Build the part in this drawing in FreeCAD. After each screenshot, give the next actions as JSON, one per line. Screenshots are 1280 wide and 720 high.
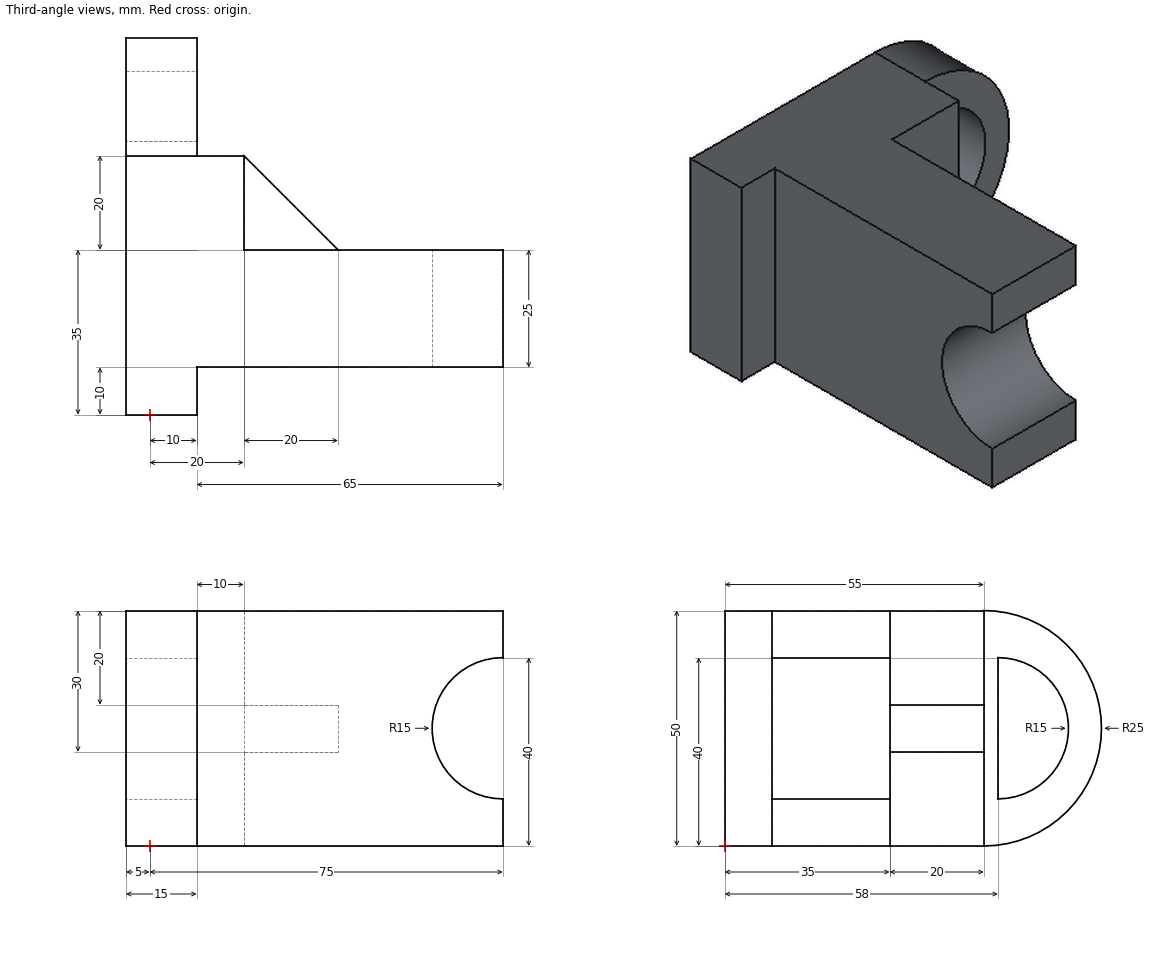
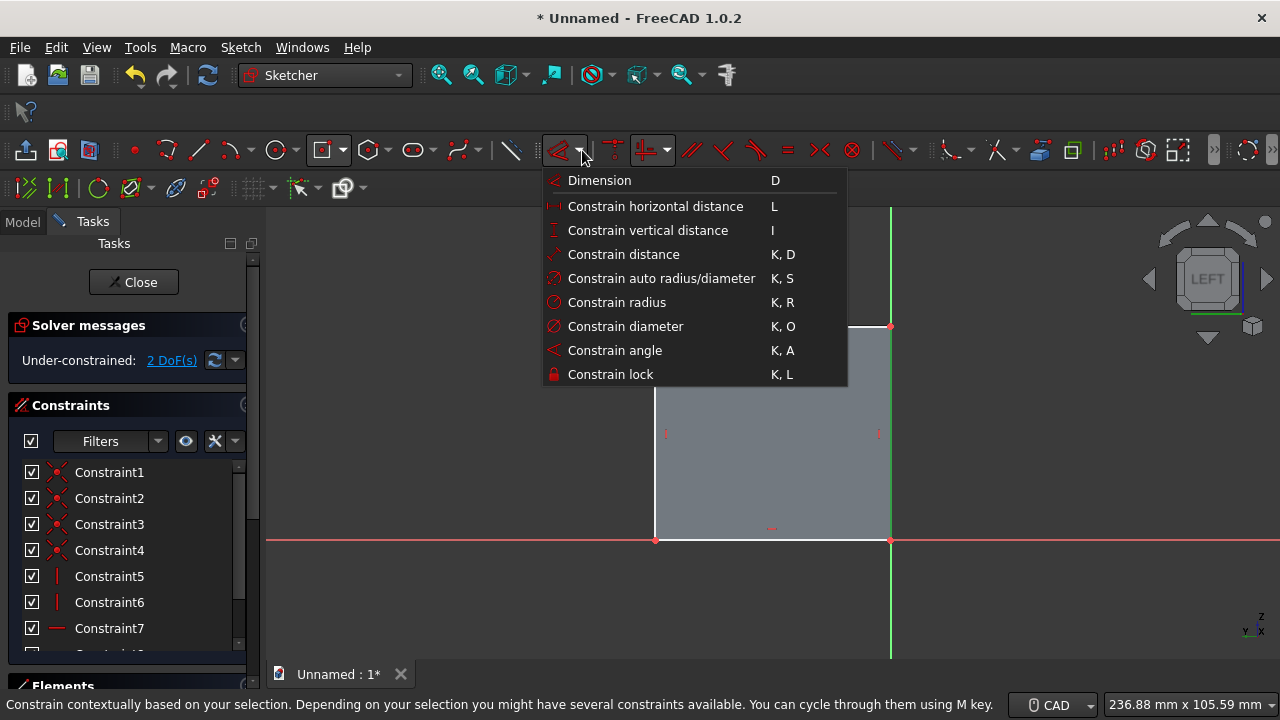
{"action": "left_click", "coordinate": [695, 230]}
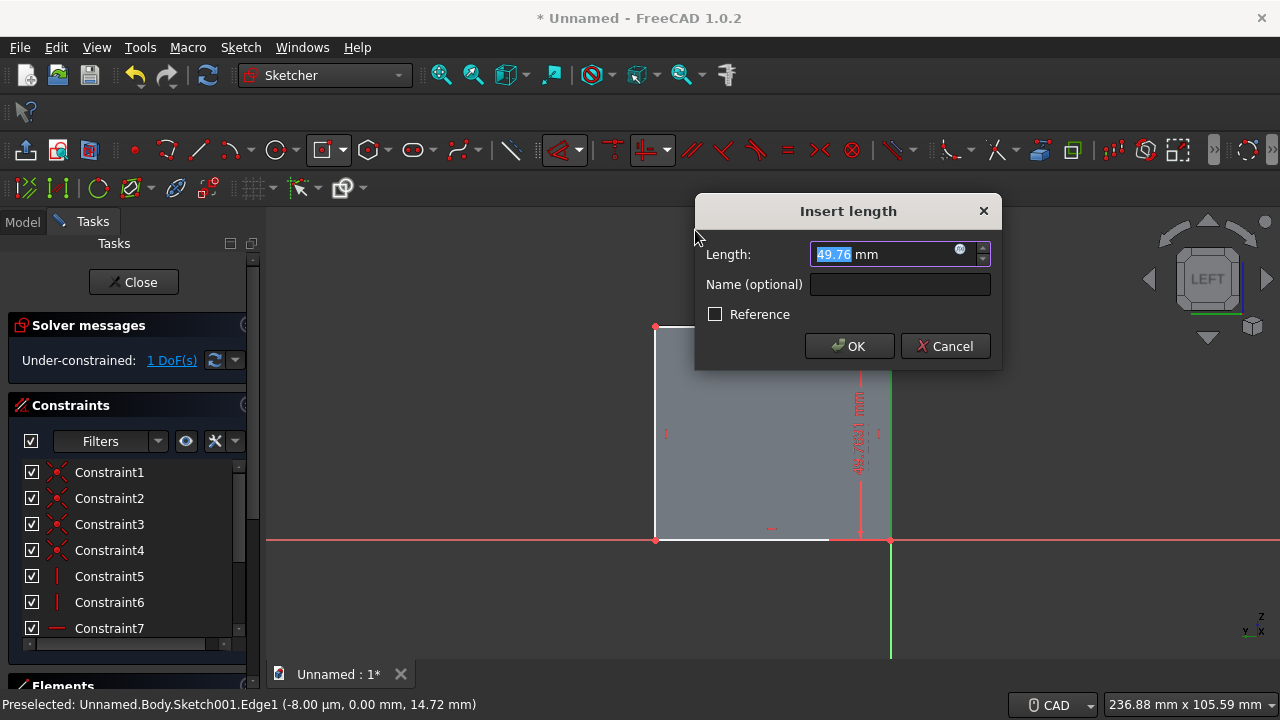
{"action": "type", "text": "50"}
{"action": "key", "text": "Return"}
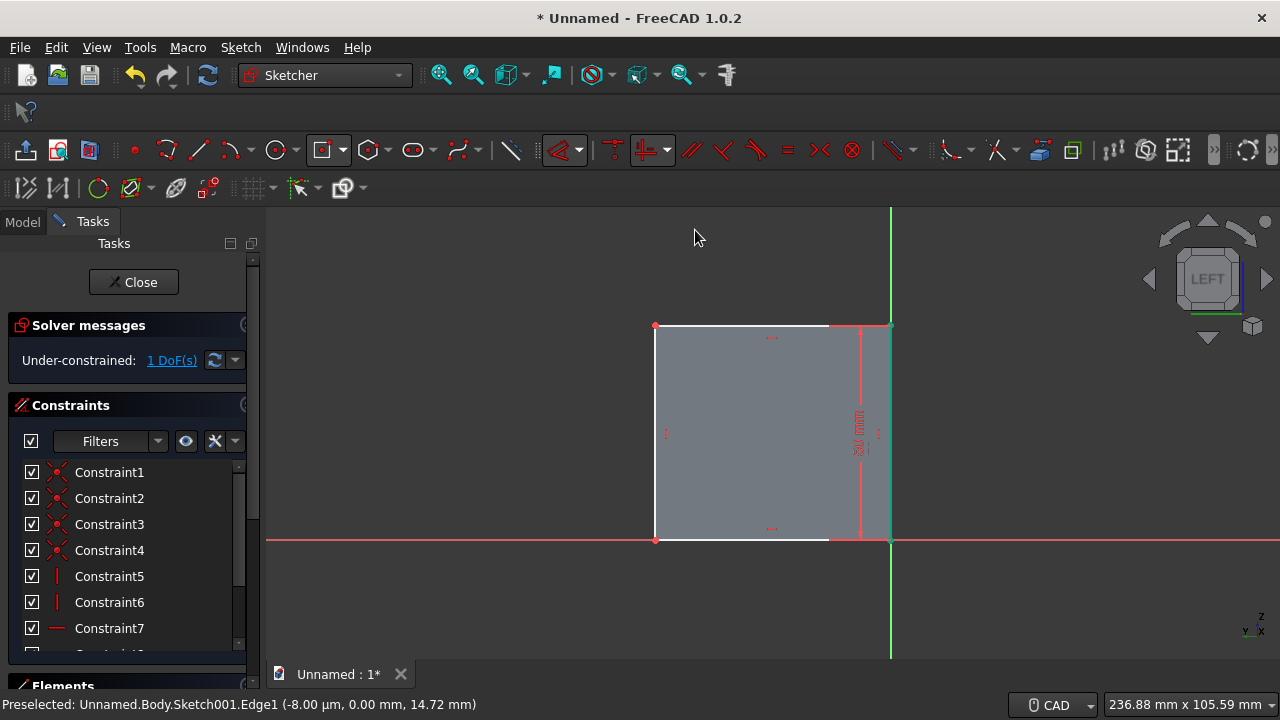
{"action": "left_click", "coordinate": [820, 326]}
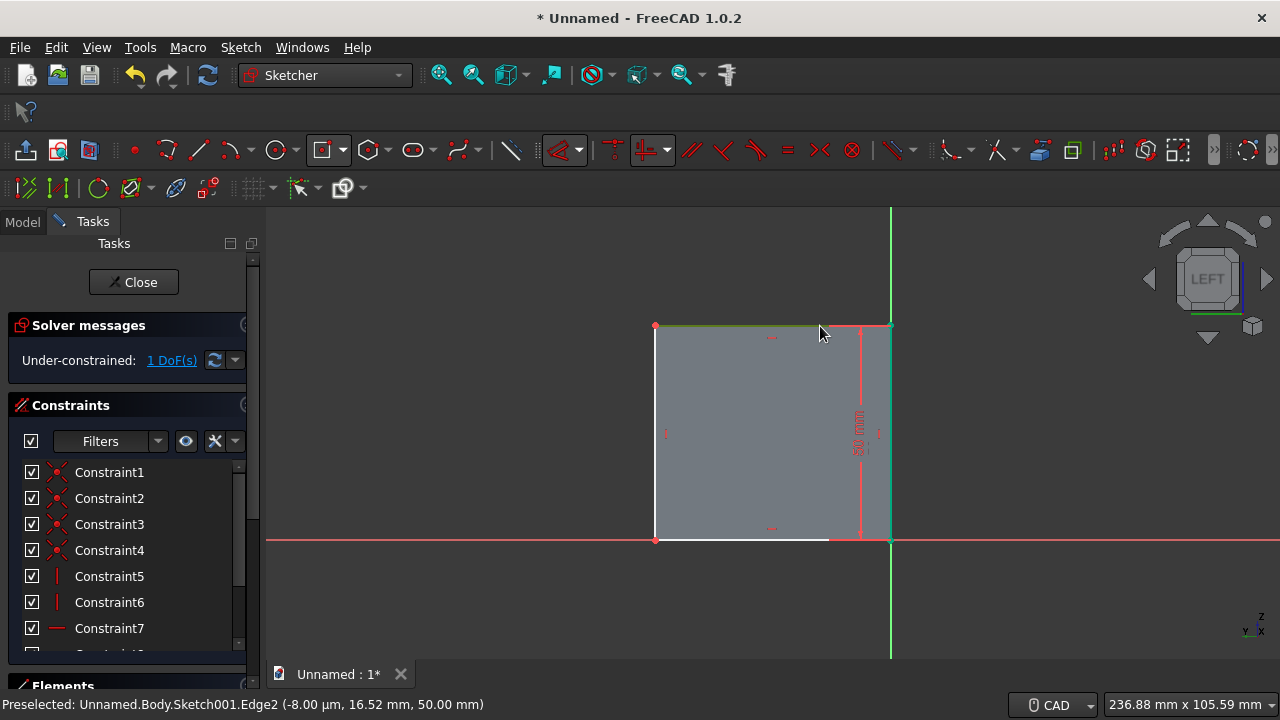
{"action": "key", "text": "l"}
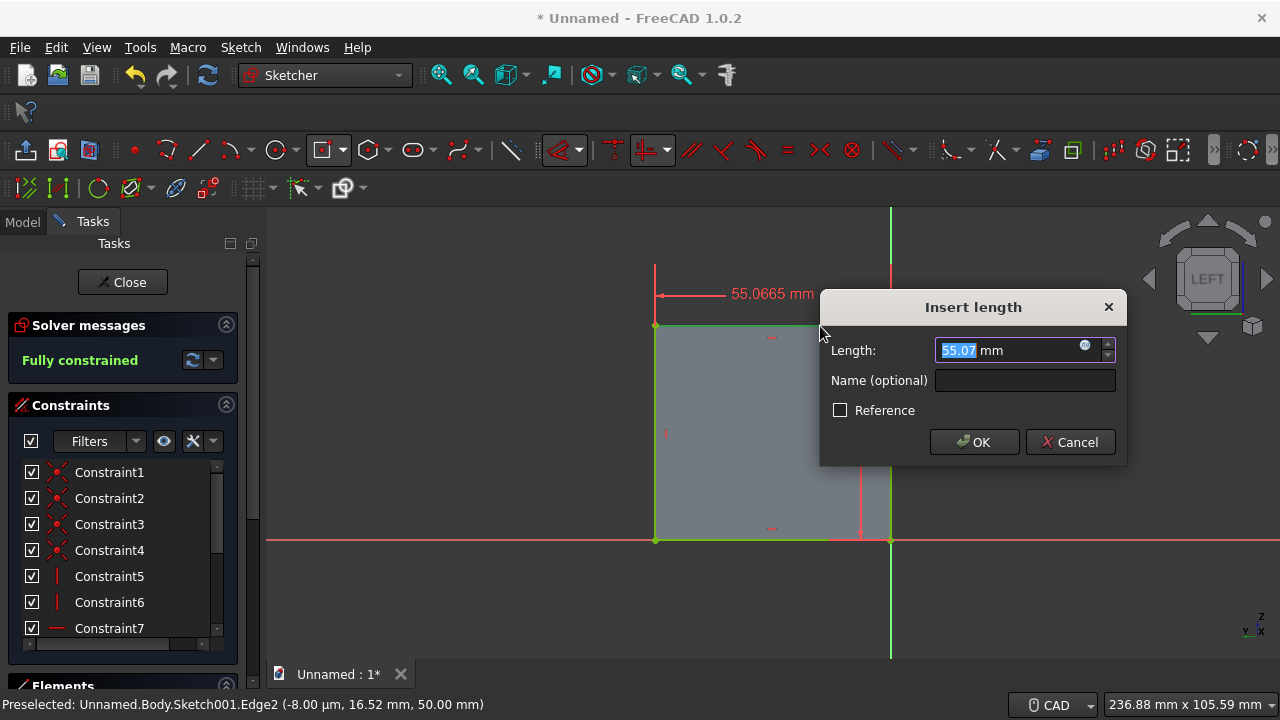
{"action": "type", "text": "55"}
{"action": "key", "text": "Return"}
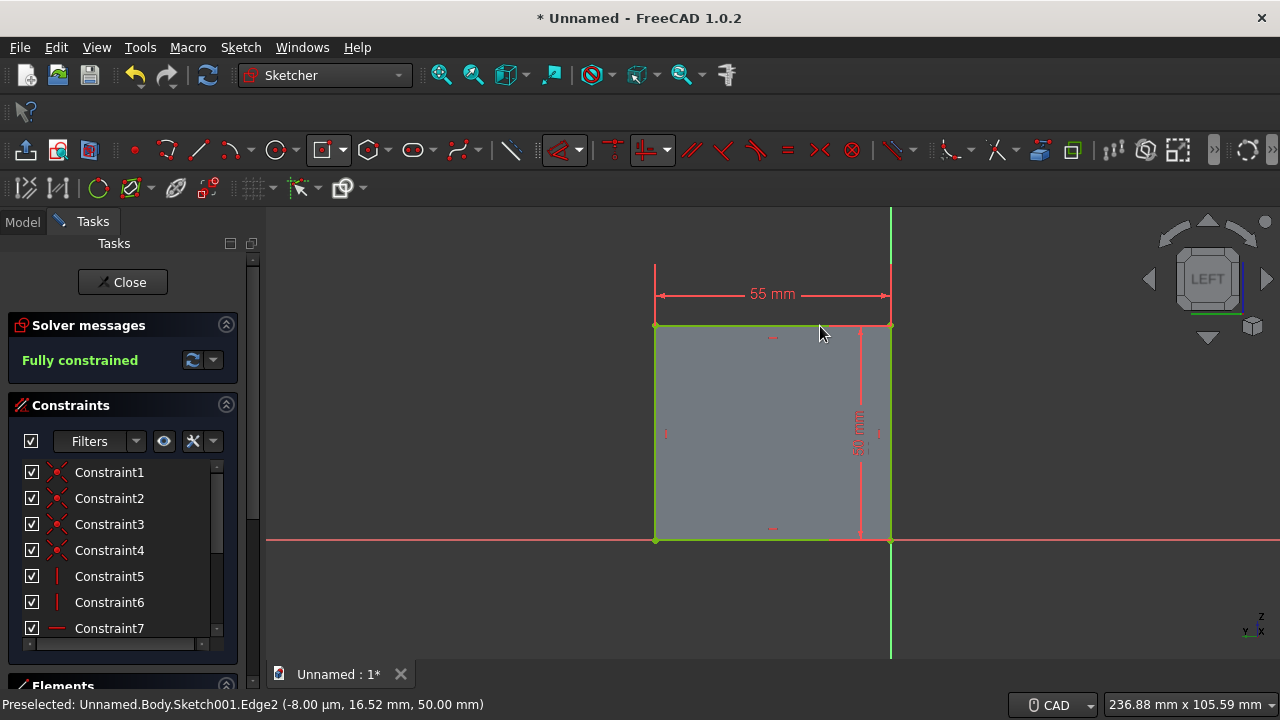
{"action": "left_click", "coordinate": [123, 282]}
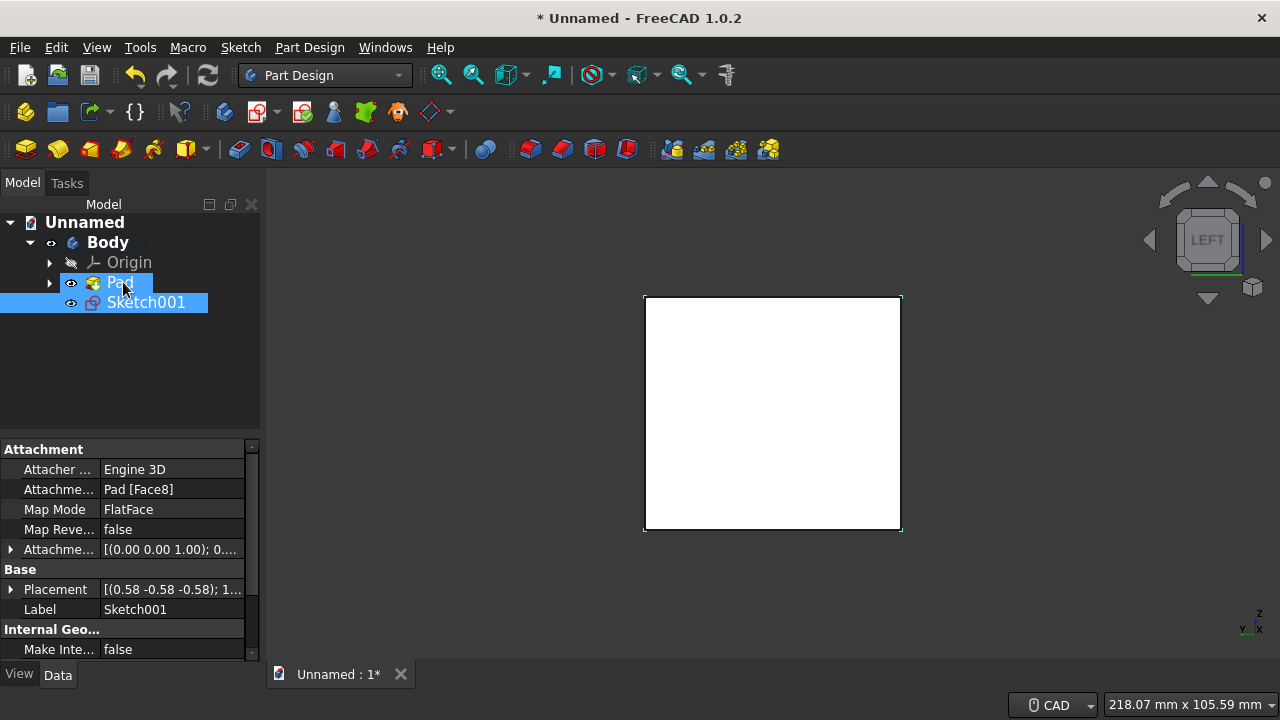
{"action": "left_click", "coordinate": [26, 150]}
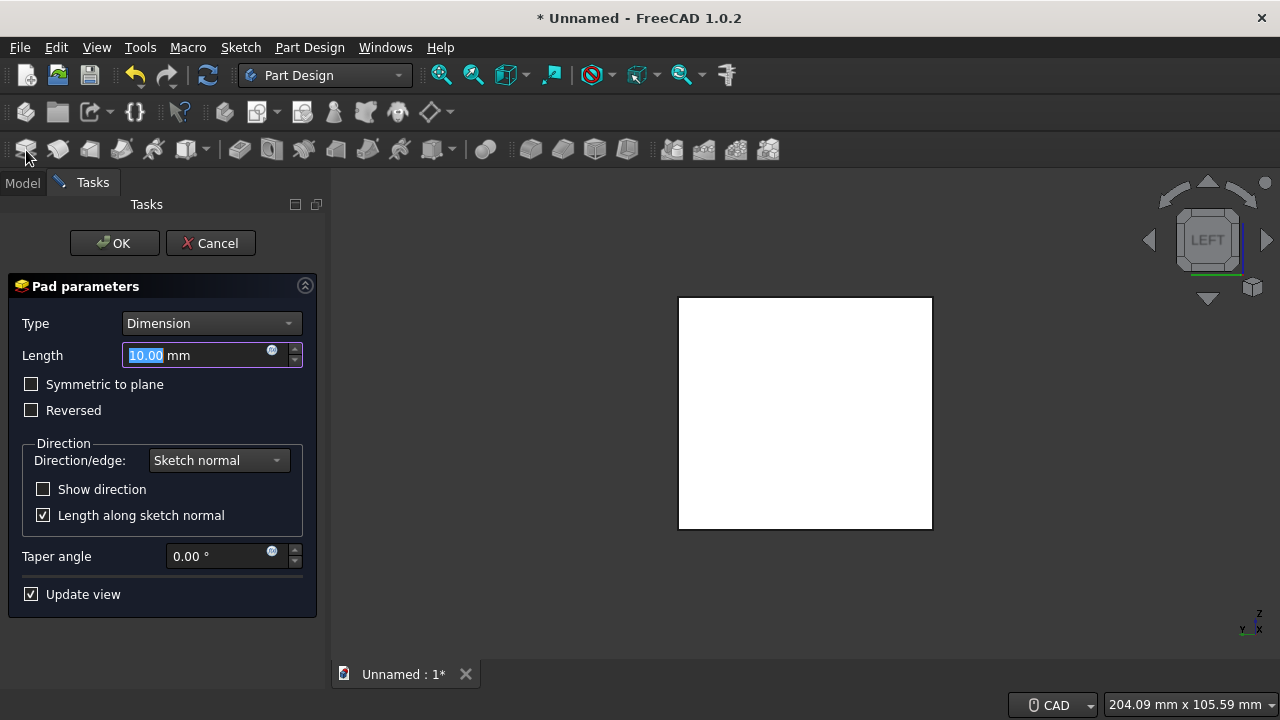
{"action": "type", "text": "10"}
{"action": "key", "text": "Tab"}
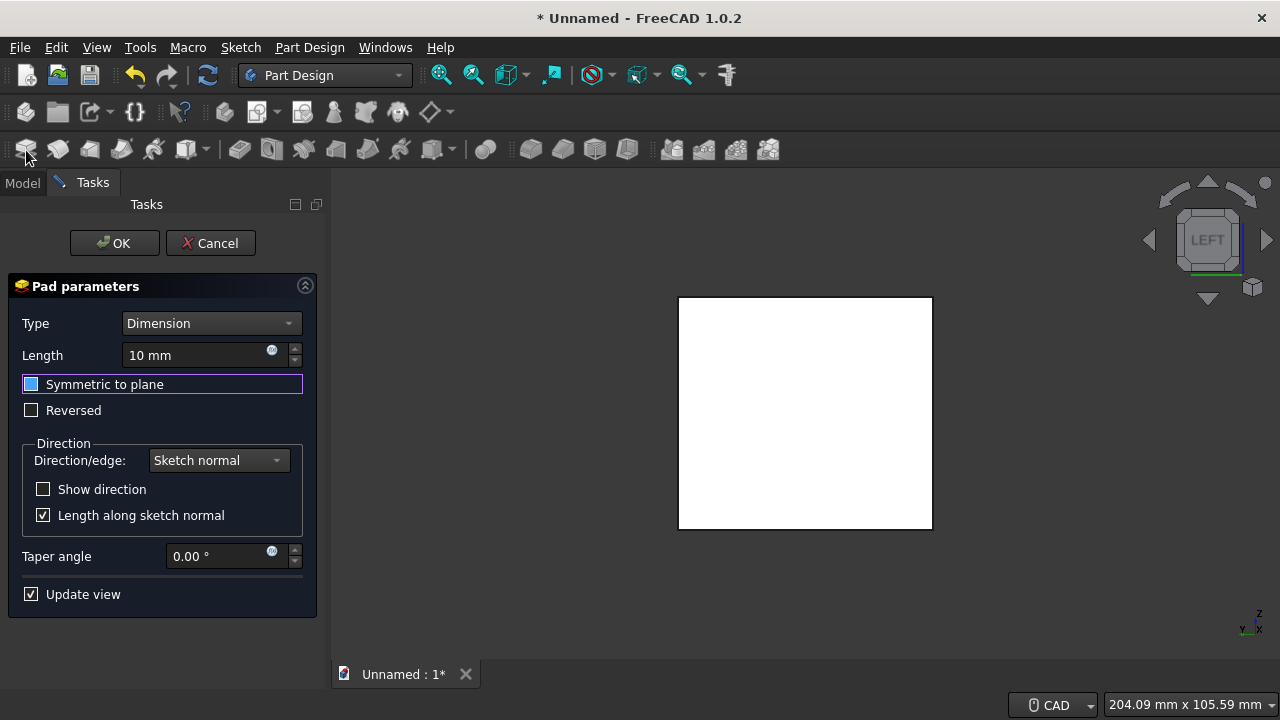
{"action": "left_click", "coordinate": [115, 243]}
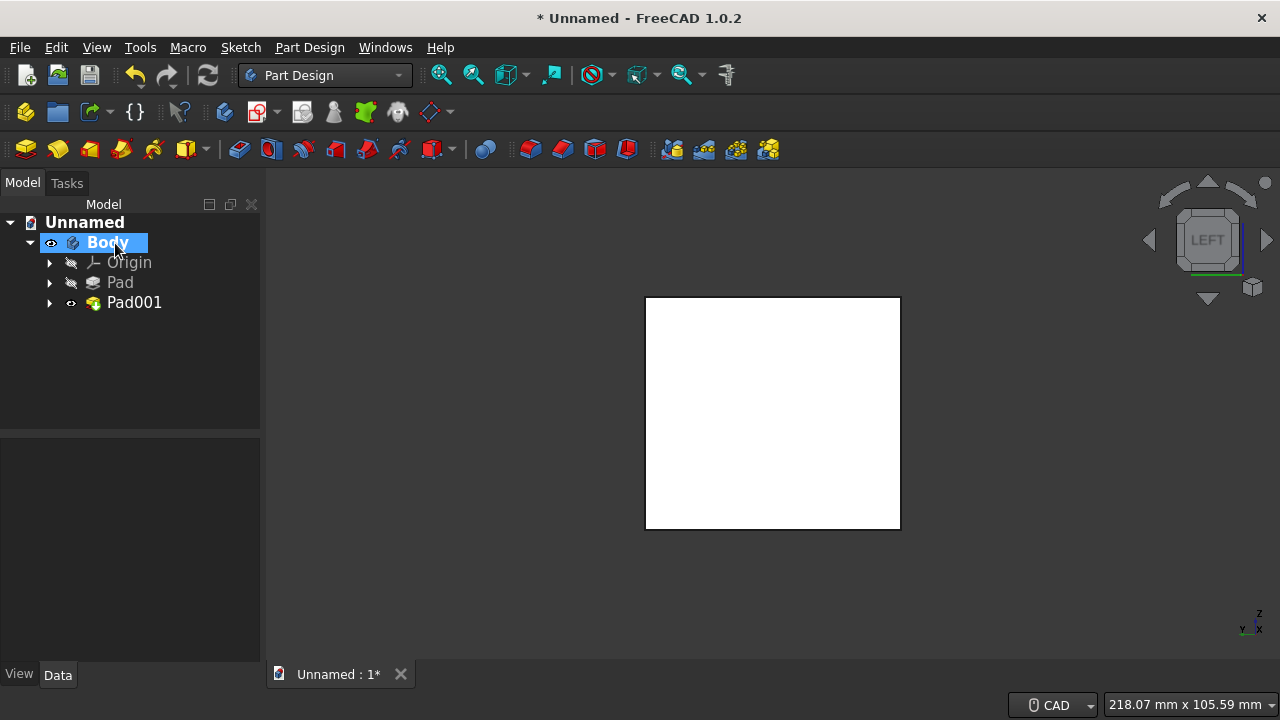
{"action": "left_click", "coordinate": [773, 413]}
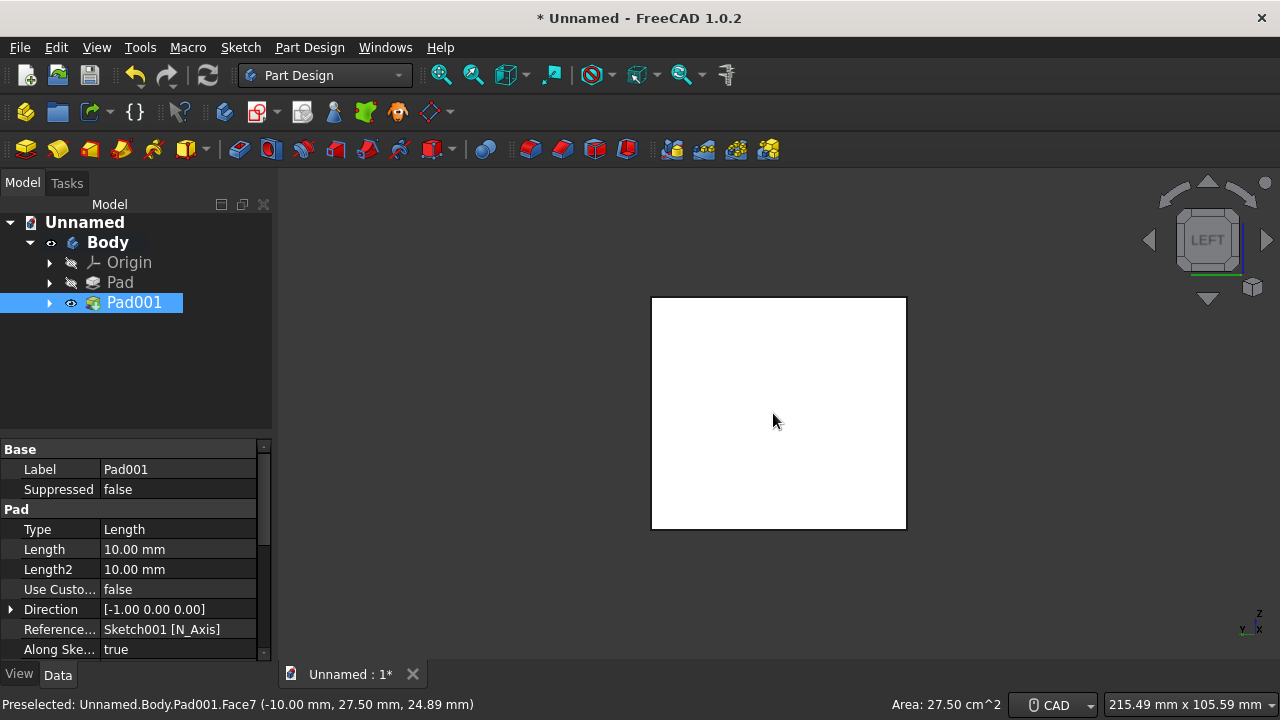
{"action": "left_click", "coordinate": [258, 112]}